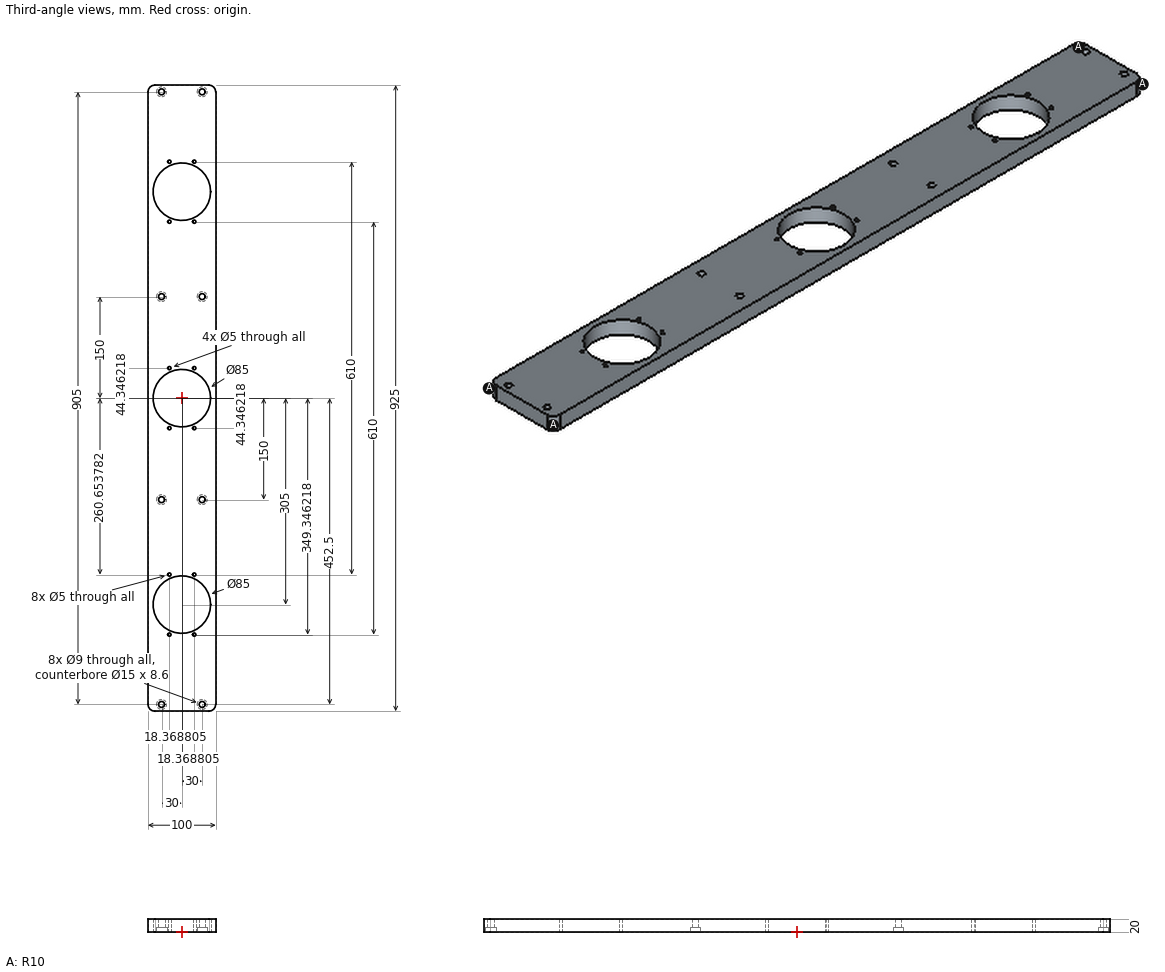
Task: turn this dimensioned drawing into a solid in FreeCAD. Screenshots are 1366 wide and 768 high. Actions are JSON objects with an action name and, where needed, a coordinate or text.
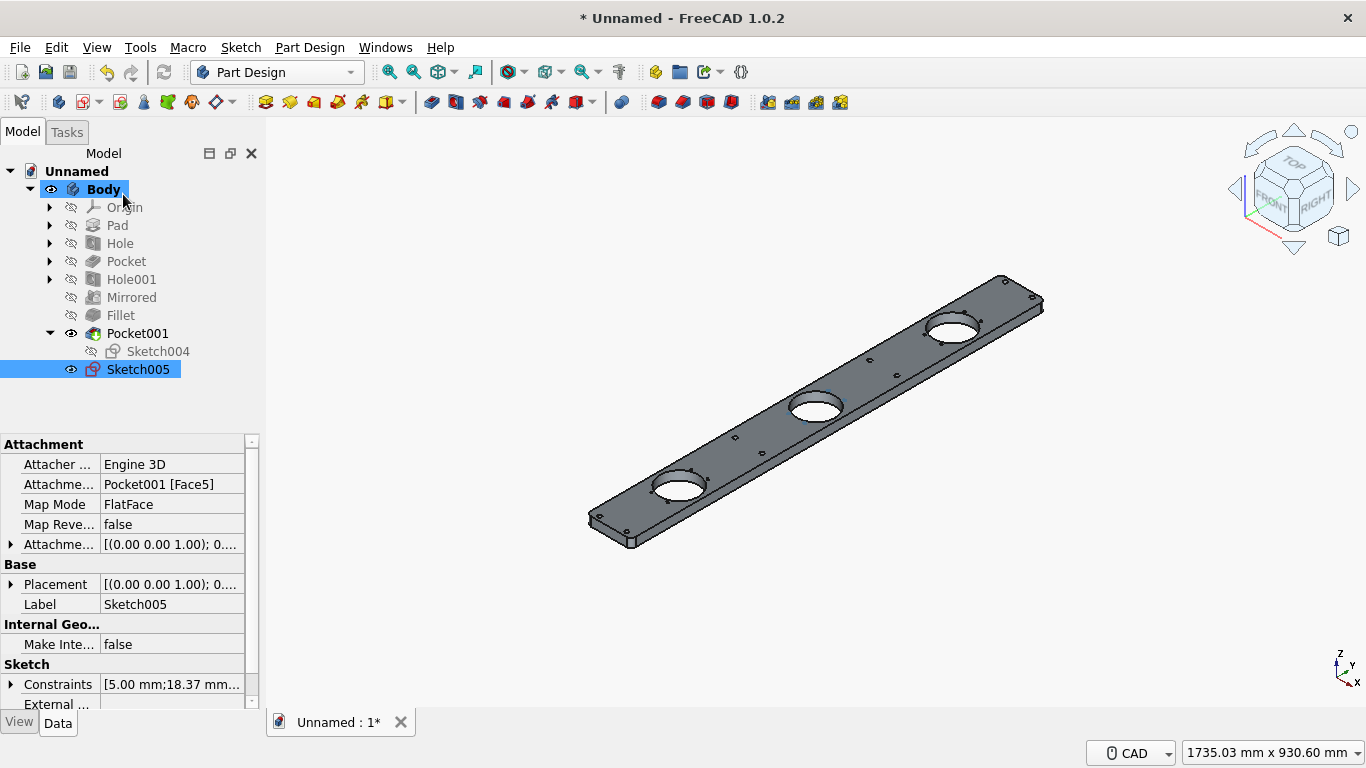
{"action": "left_click", "coordinate": [456, 102]}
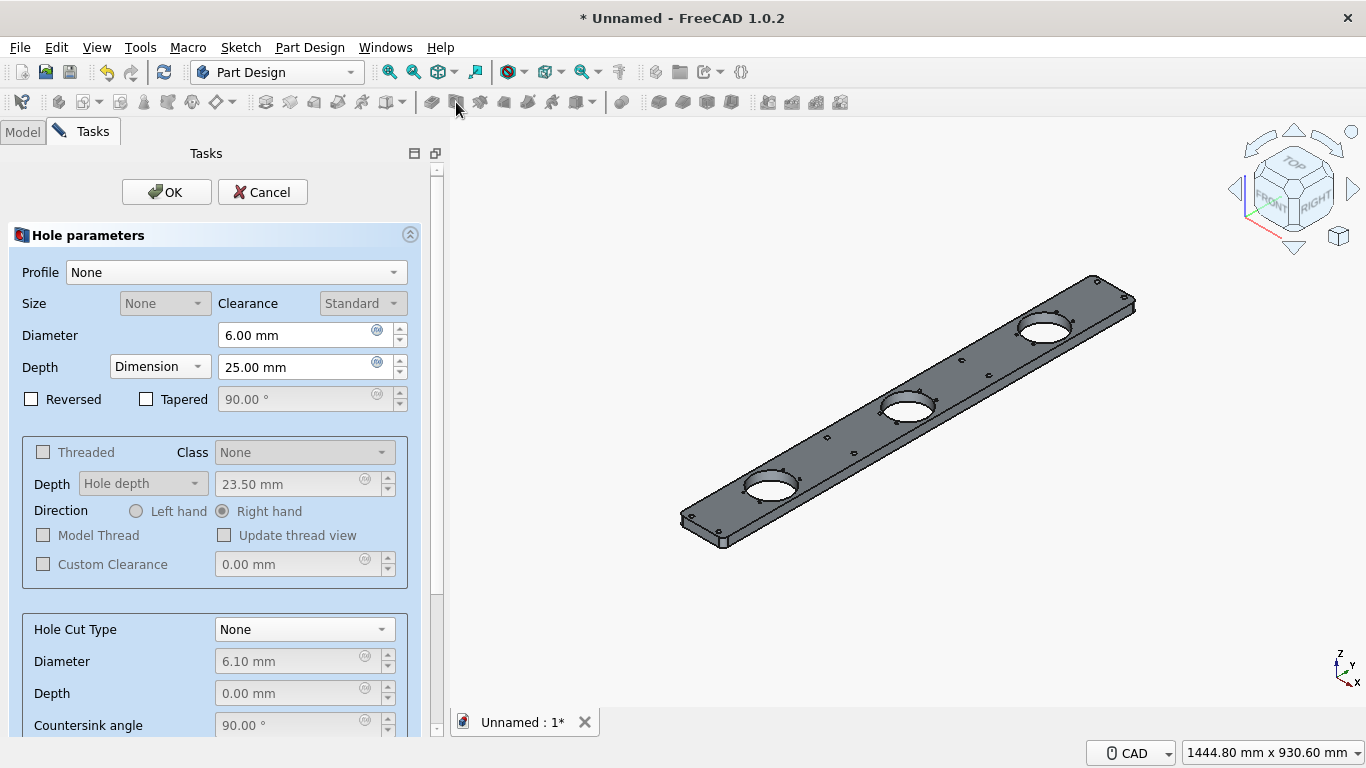
{"action": "triple_click", "coordinate": [305, 335]}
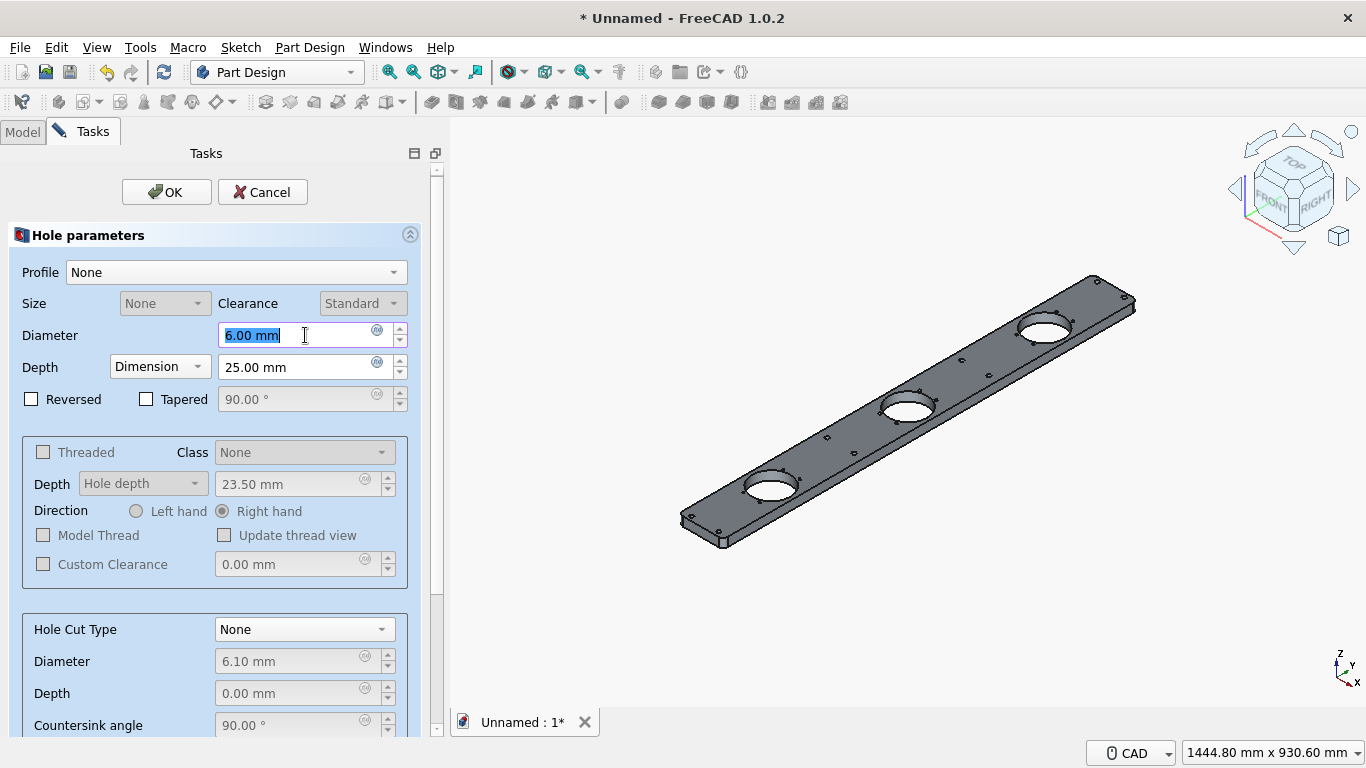
{"action": "type", "text": "5"}
{"action": "key", "text": "Tab"}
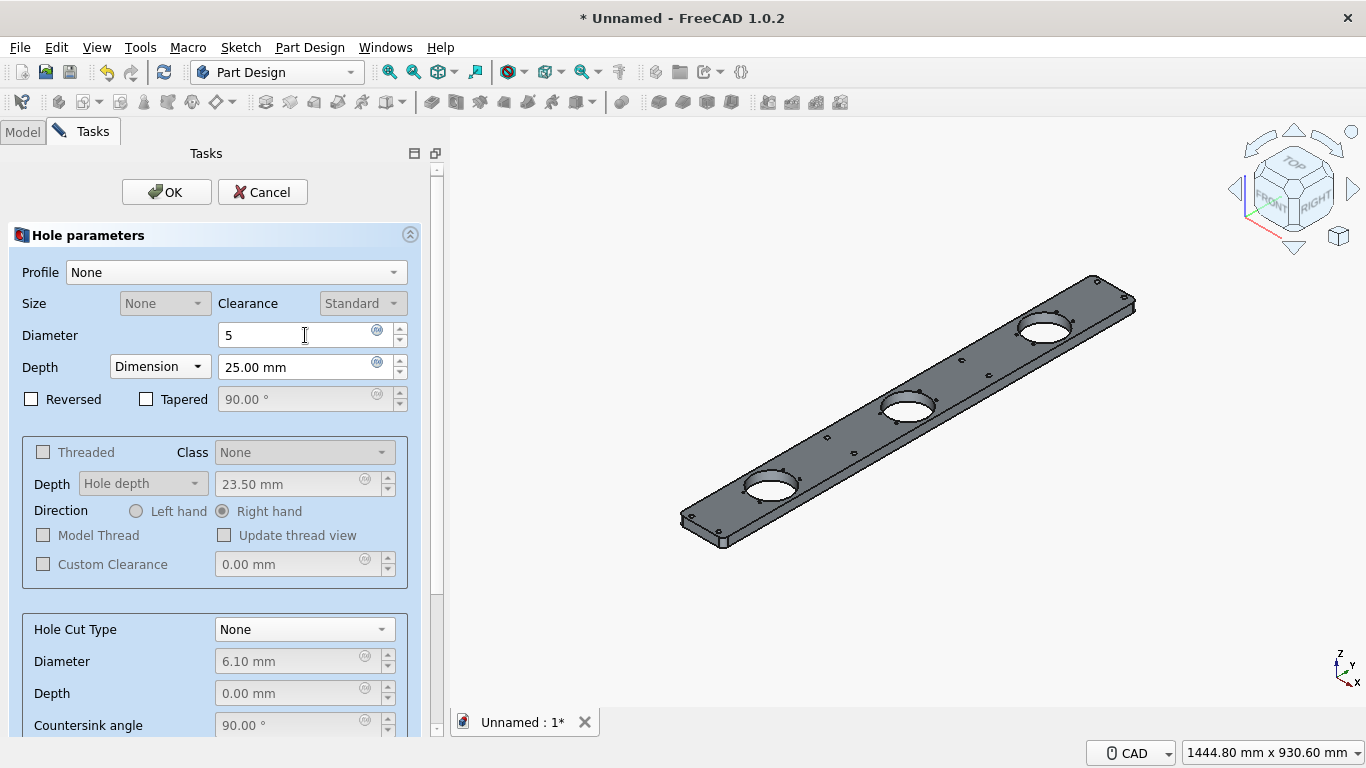
{"action": "left_click", "coordinate": [161, 366]}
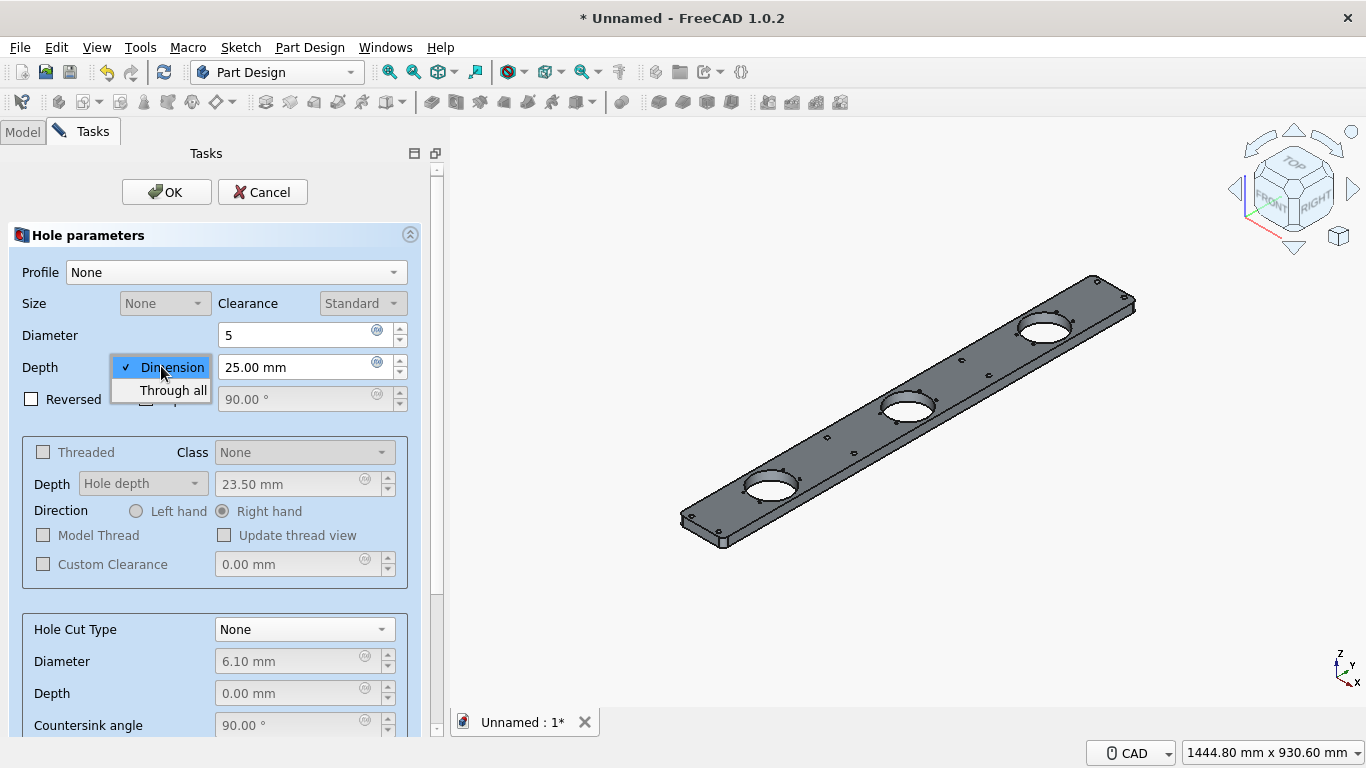
{"action": "left_click", "coordinate": [160, 390]}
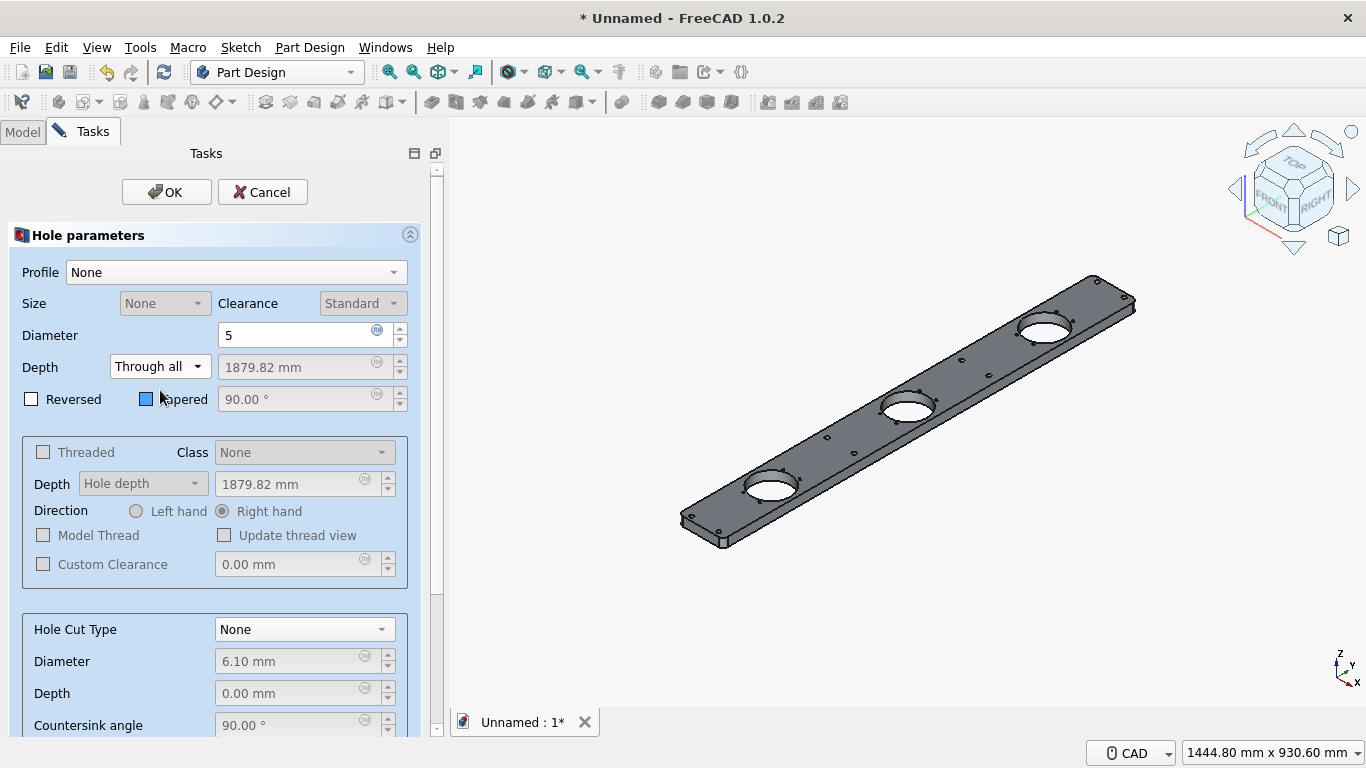
{"action": "left_click", "coordinate": [167, 192]}